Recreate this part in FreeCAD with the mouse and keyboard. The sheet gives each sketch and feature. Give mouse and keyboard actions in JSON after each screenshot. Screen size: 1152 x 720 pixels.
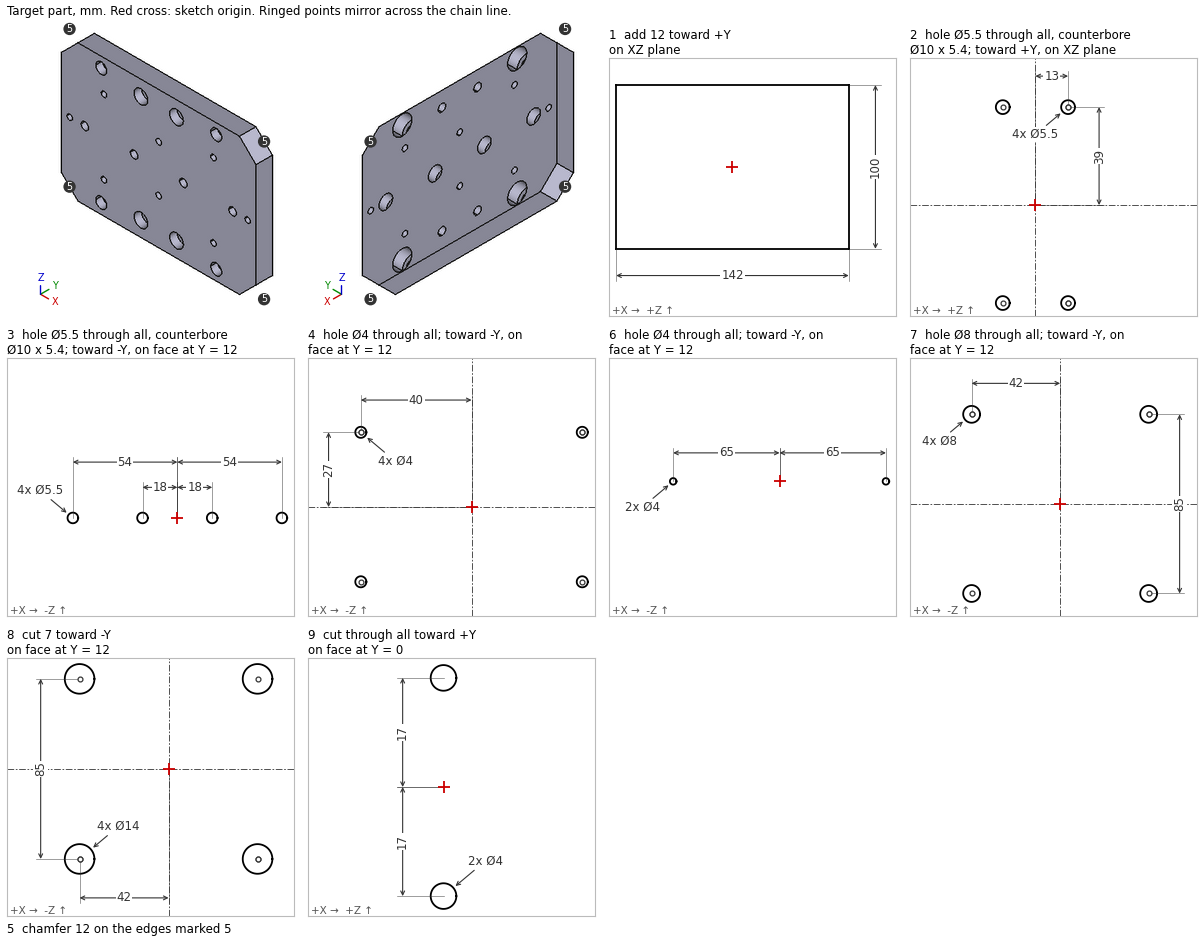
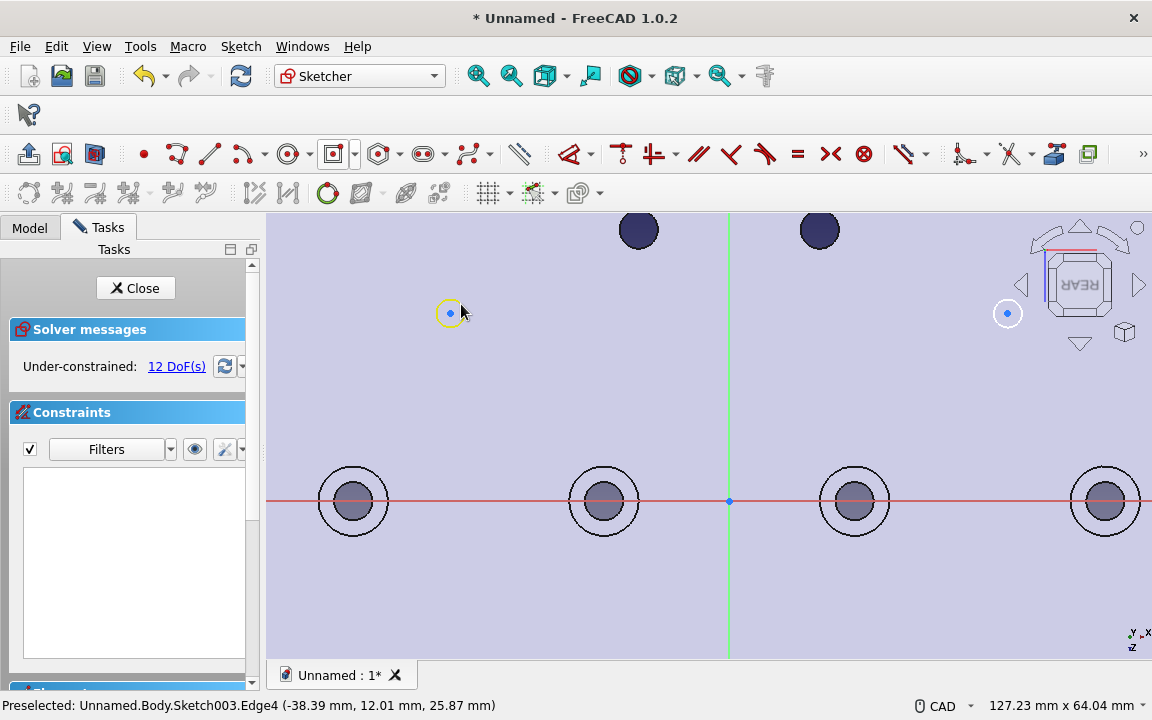
{"action": "left_click", "coordinate": [460, 304]}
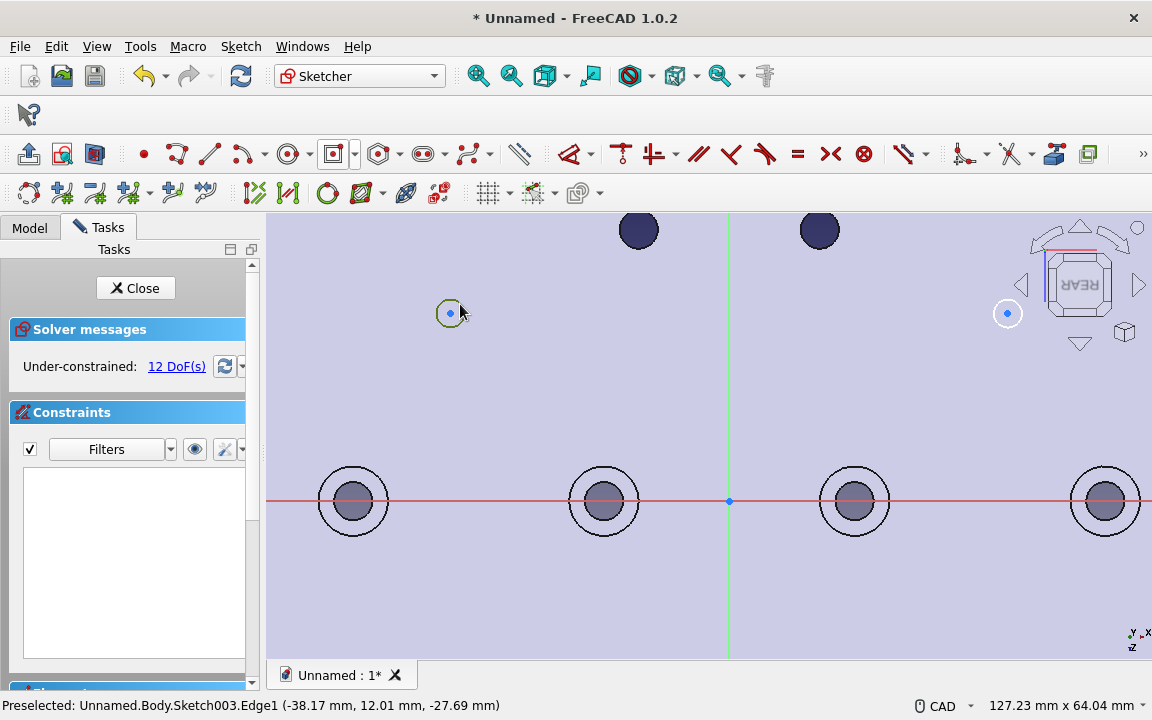
{"action": "scroll", "coordinate": [460, 304], "scroll_direction": "down", "scroll_amount": 2}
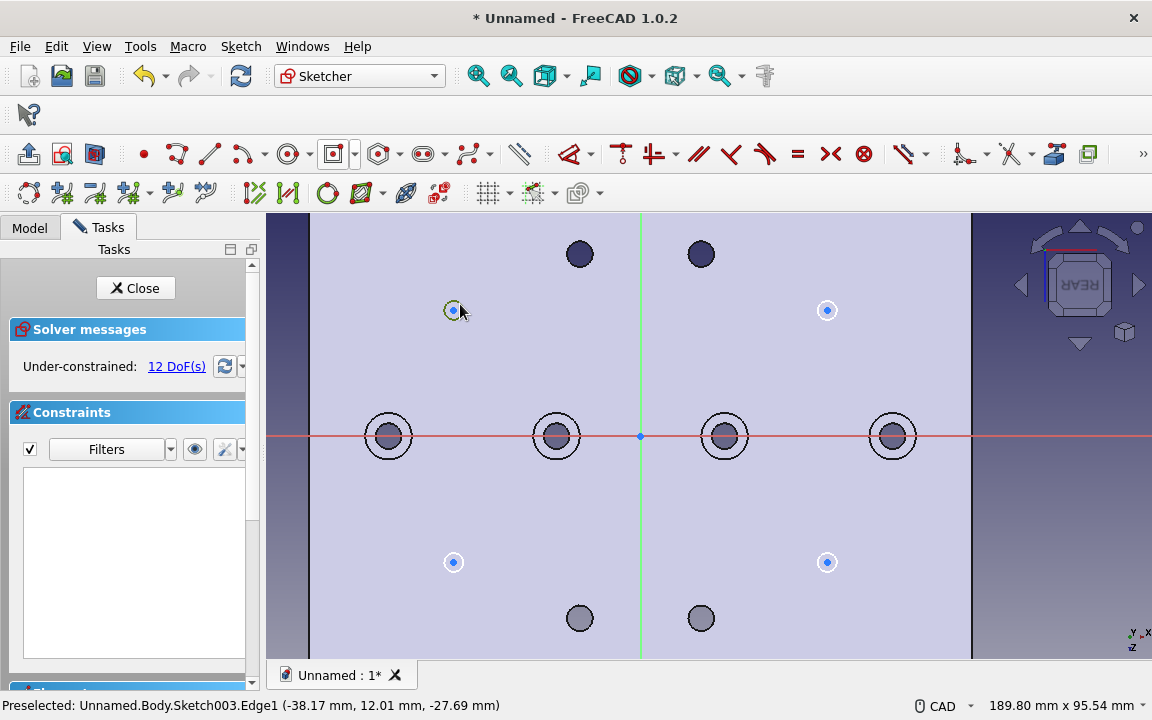
{"action": "scroll", "coordinate": [834, 304], "scroll_direction": "up", "scroll_amount": 2}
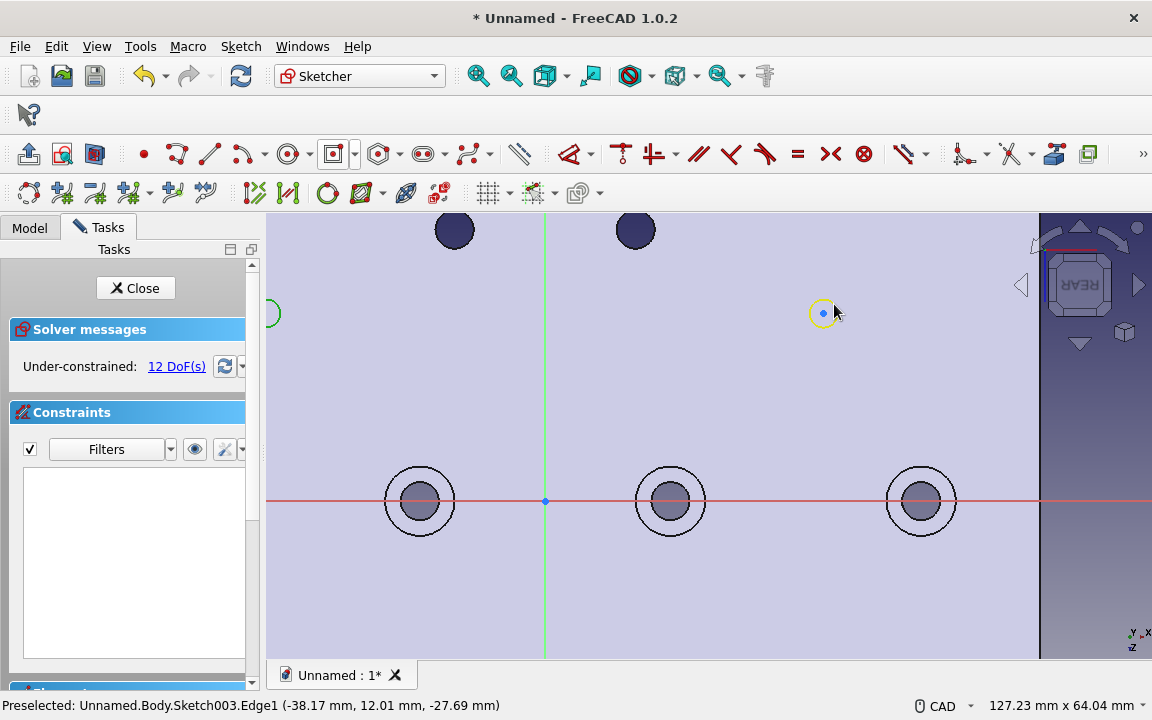
{"action": "left_click", "coordinate": [834, 304]}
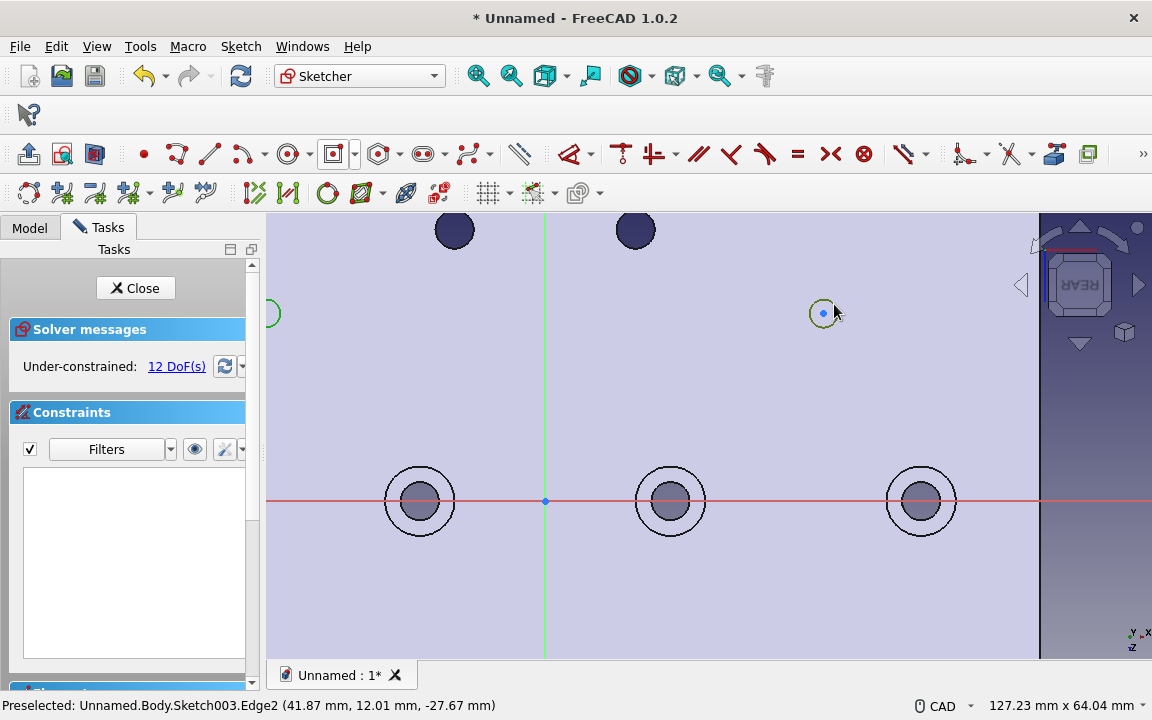
{"action": "scroll", "coordinate": [834, 304], "scroll_direction": "down", "scroll_amount": 2}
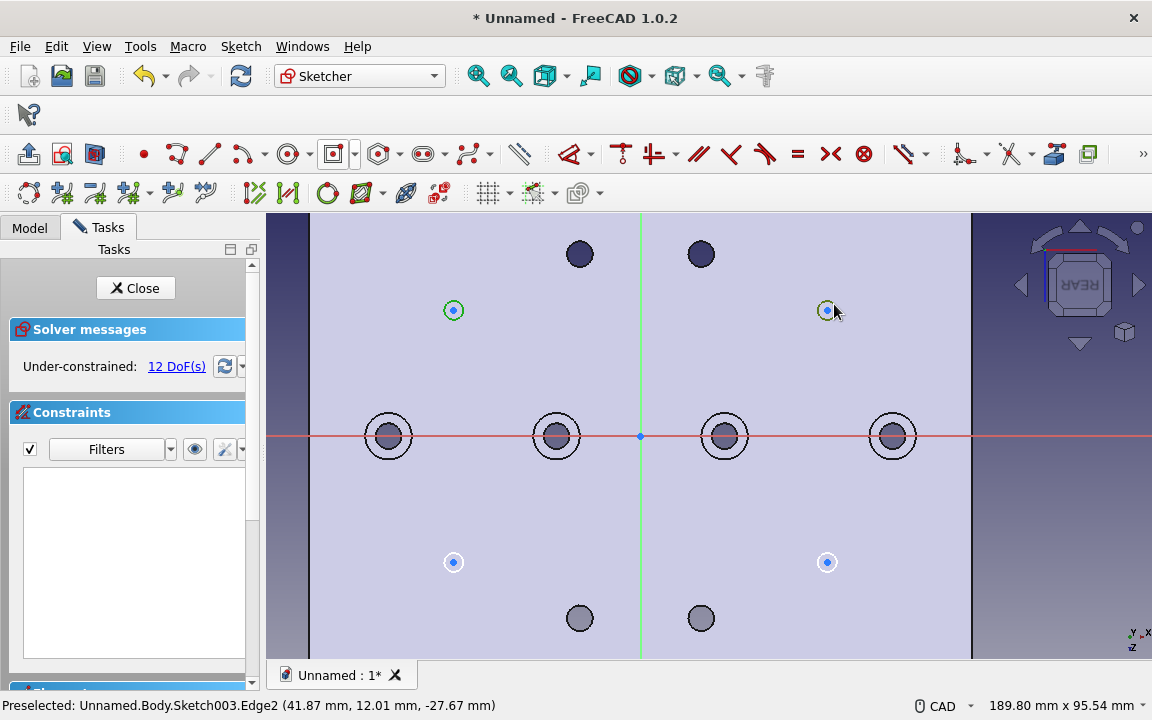
{"action": "scroll", "coordinate": [834, 556], "scroll_direction": "up", "scroll_amount": 2}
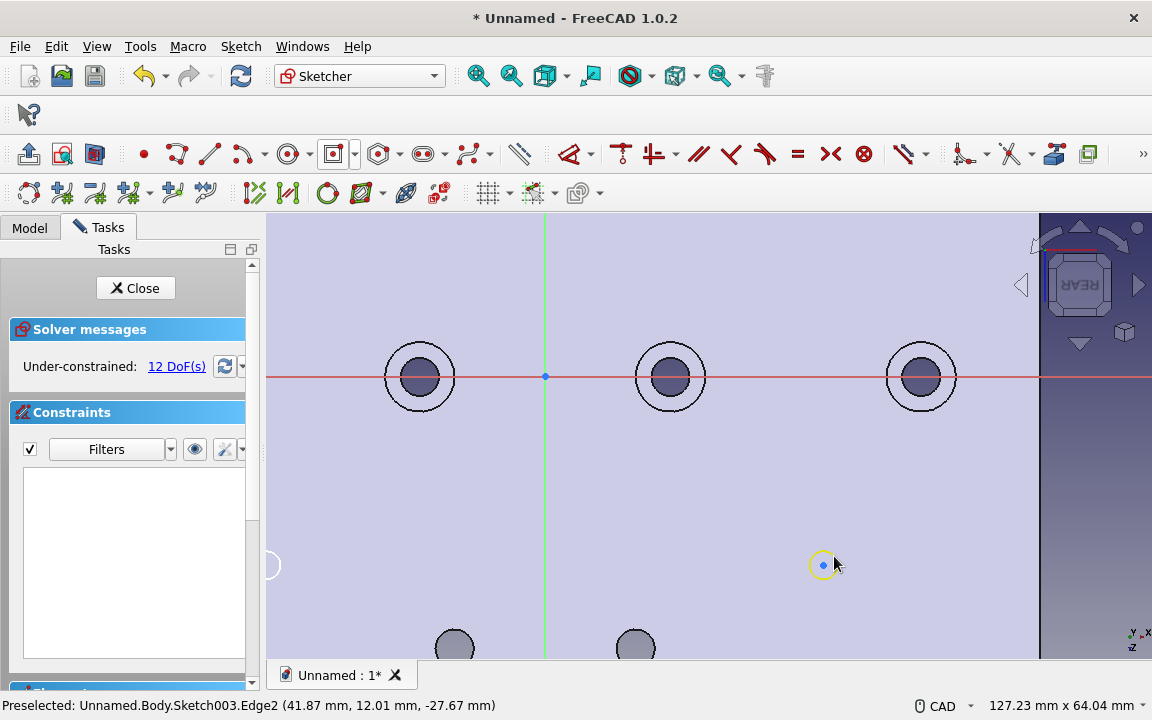
{"action": "left_click", "coordinate": [834, 555]}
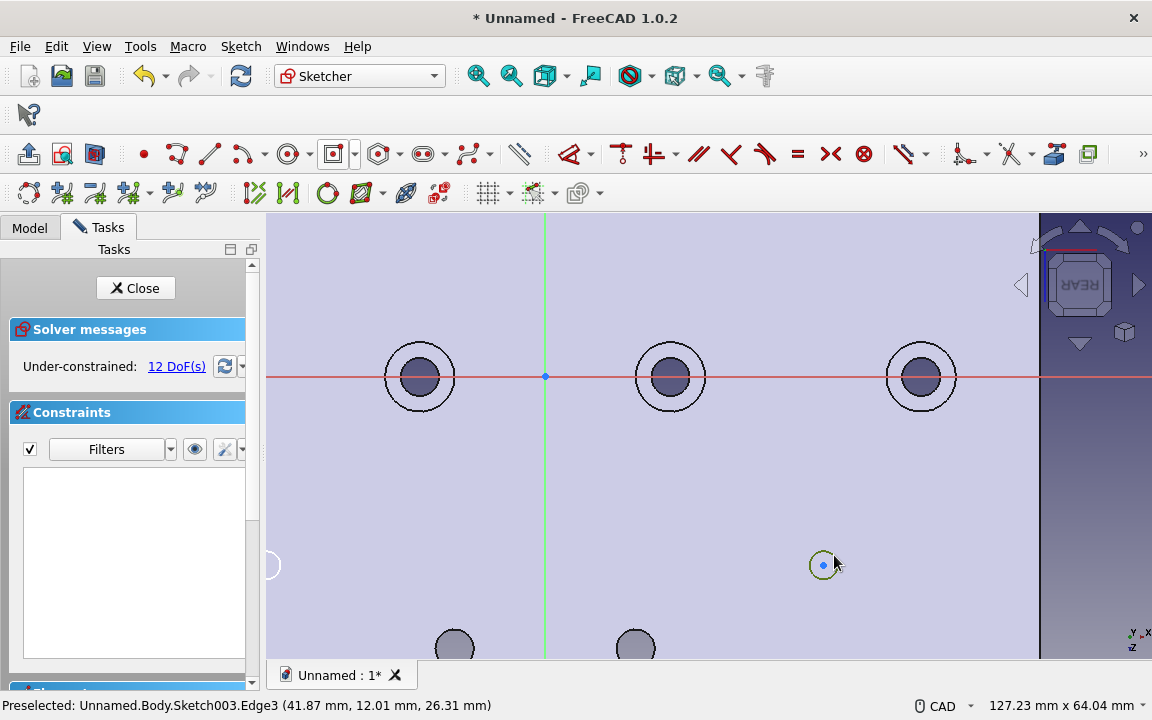
{"action": "scroll", "coordinate": [834, 556], "scroll_direction": "down", "scroll_amount": 2}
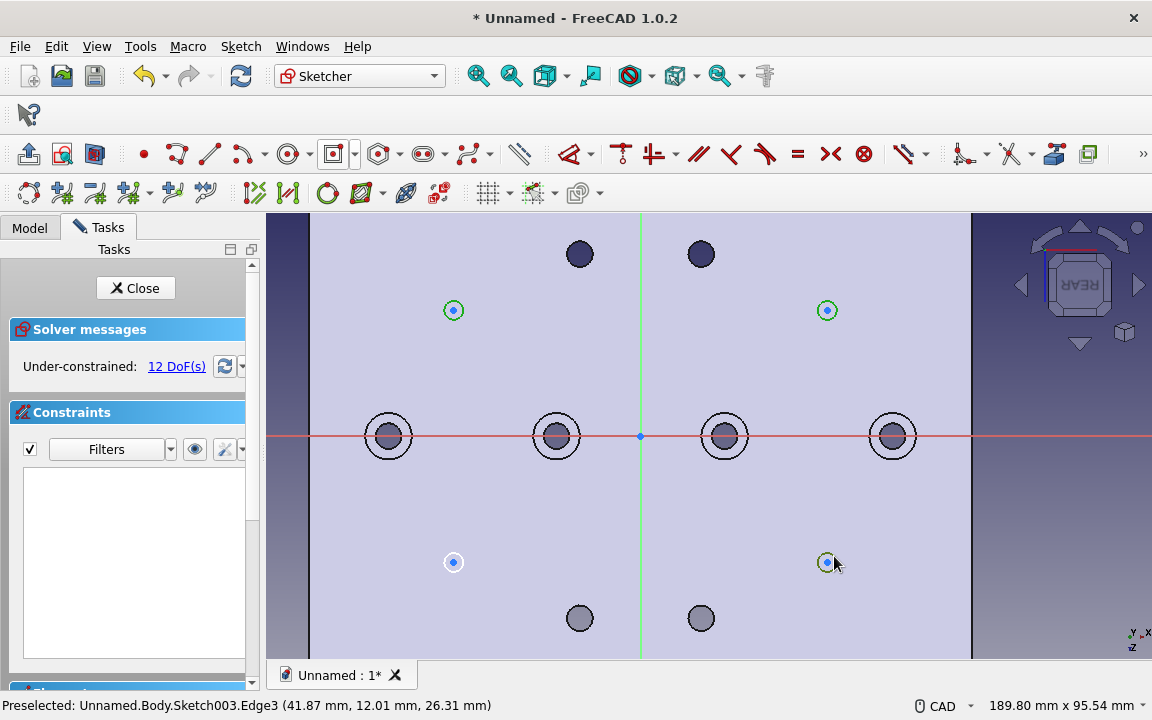
{"action": "scroll", "coordinate": [460, 556], "scroll_direction": "up", "scroll_amount": 2}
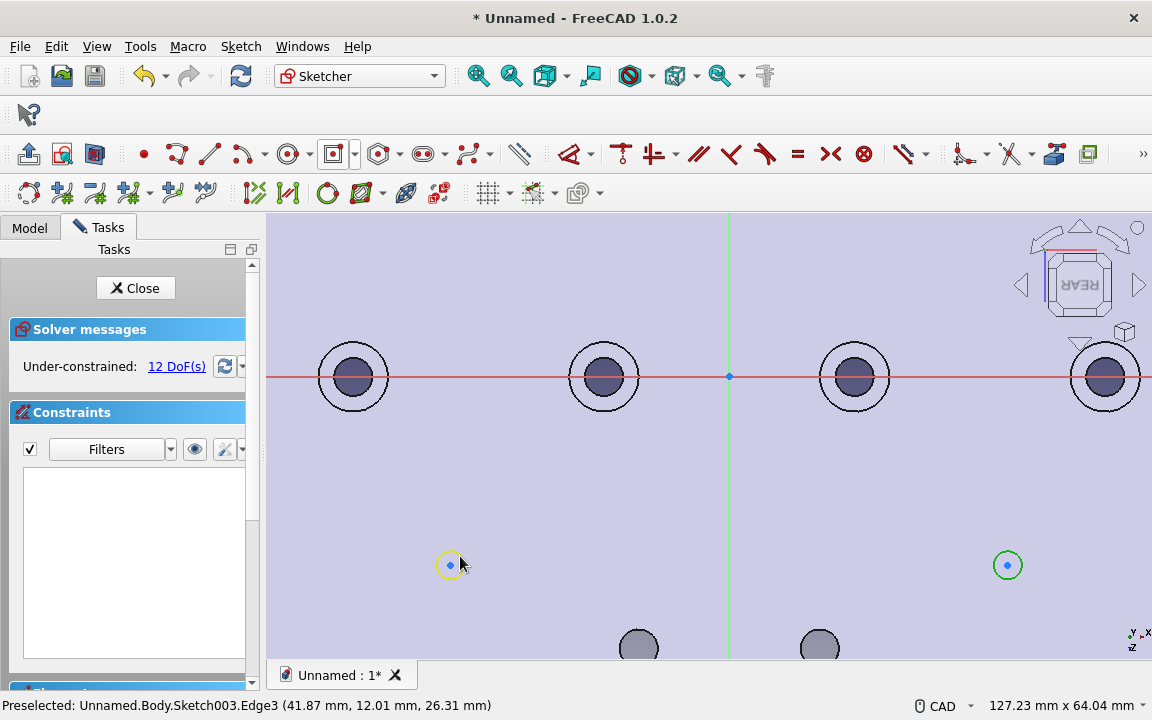
{"action": "left_click", "coordinate": [460, 555]}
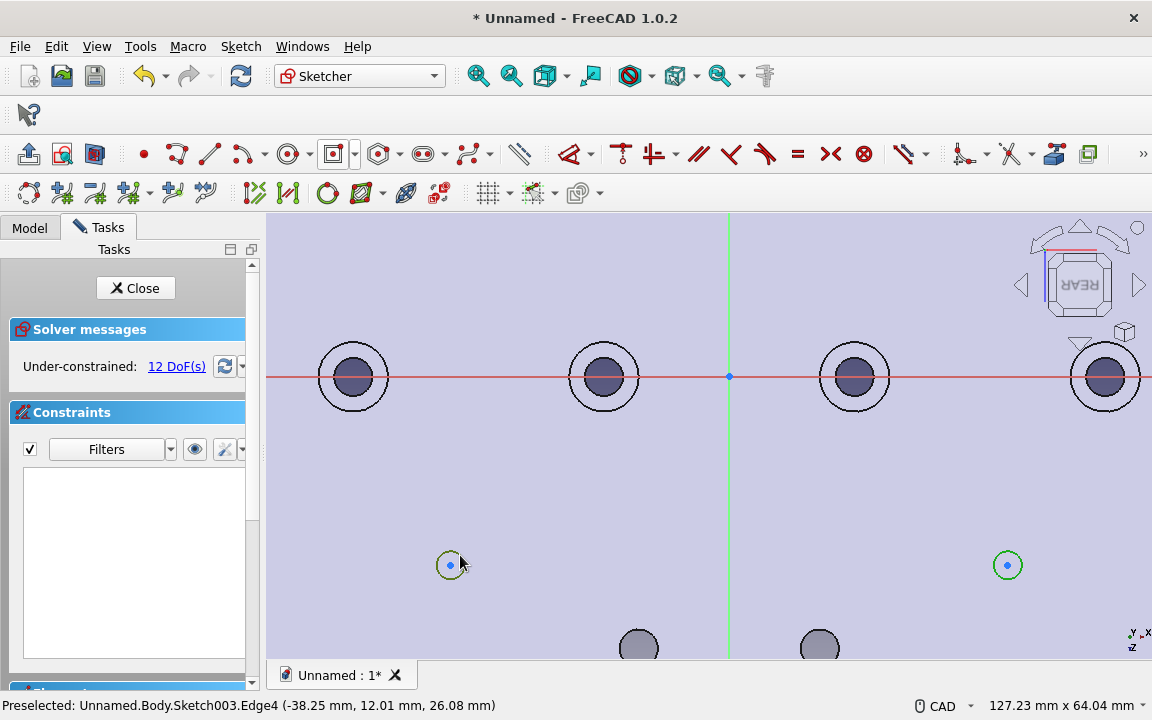
{"action": "left_click", "coordinate": [798, 154]}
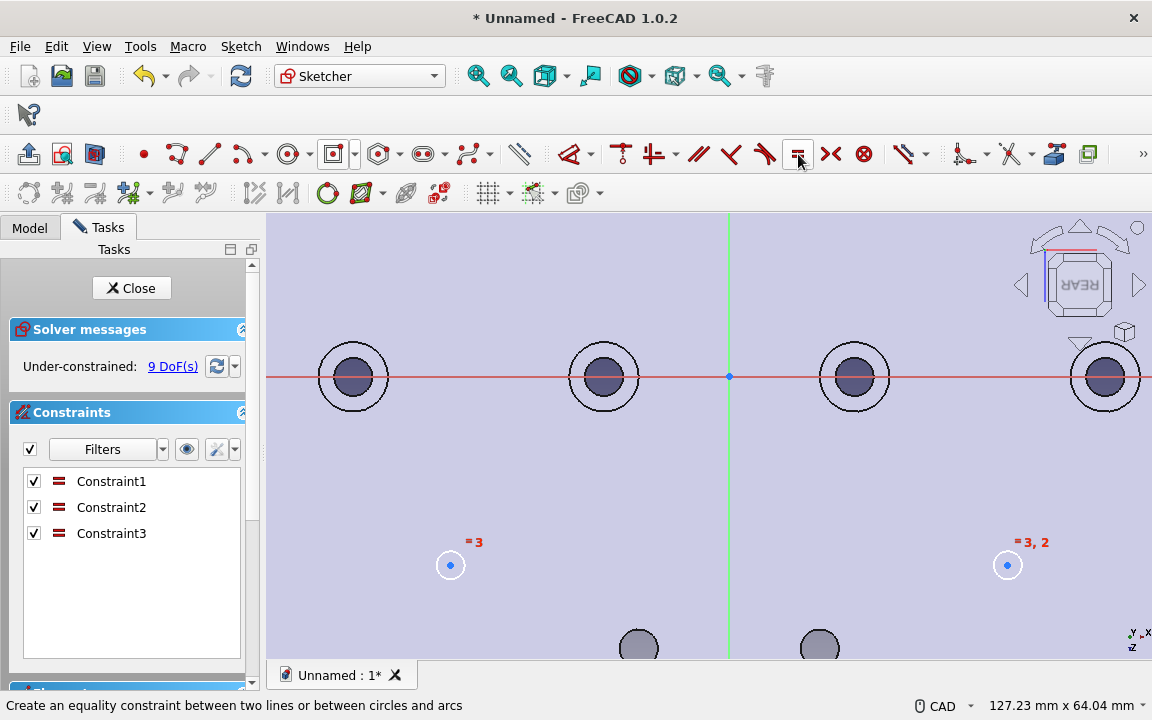
{"action": "scroll", "coordinate": [460, 556], "scroll_direction": "down", "scroll_amount": 2}